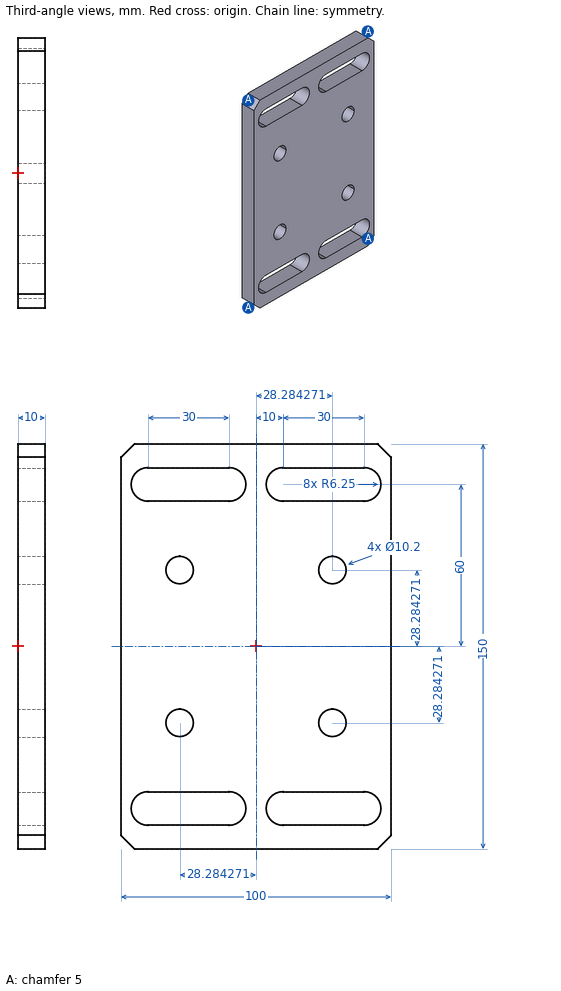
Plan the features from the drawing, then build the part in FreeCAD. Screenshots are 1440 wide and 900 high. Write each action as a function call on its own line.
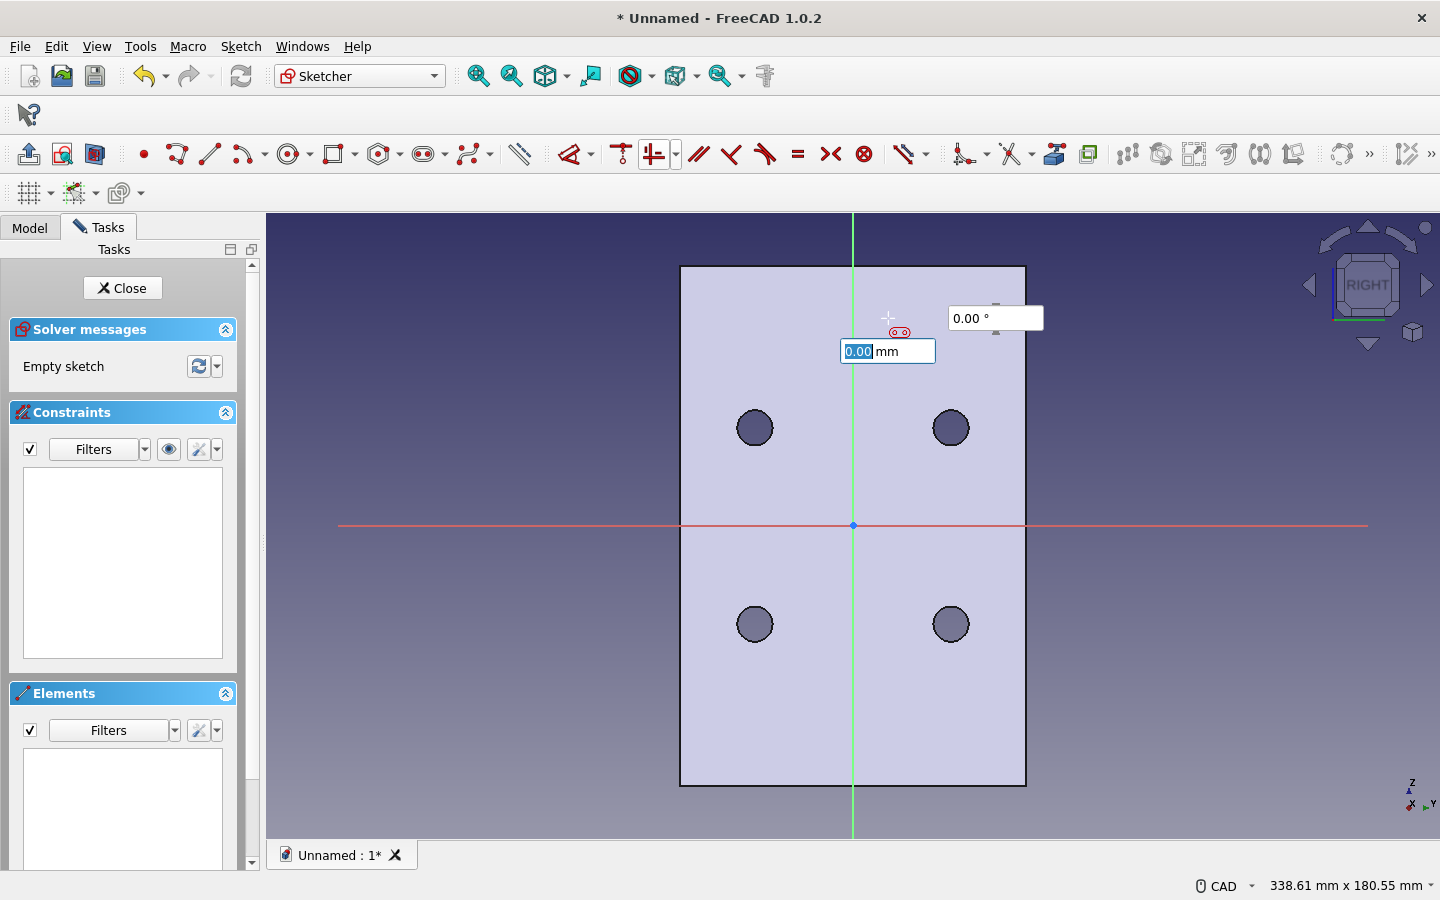
click(992, 318)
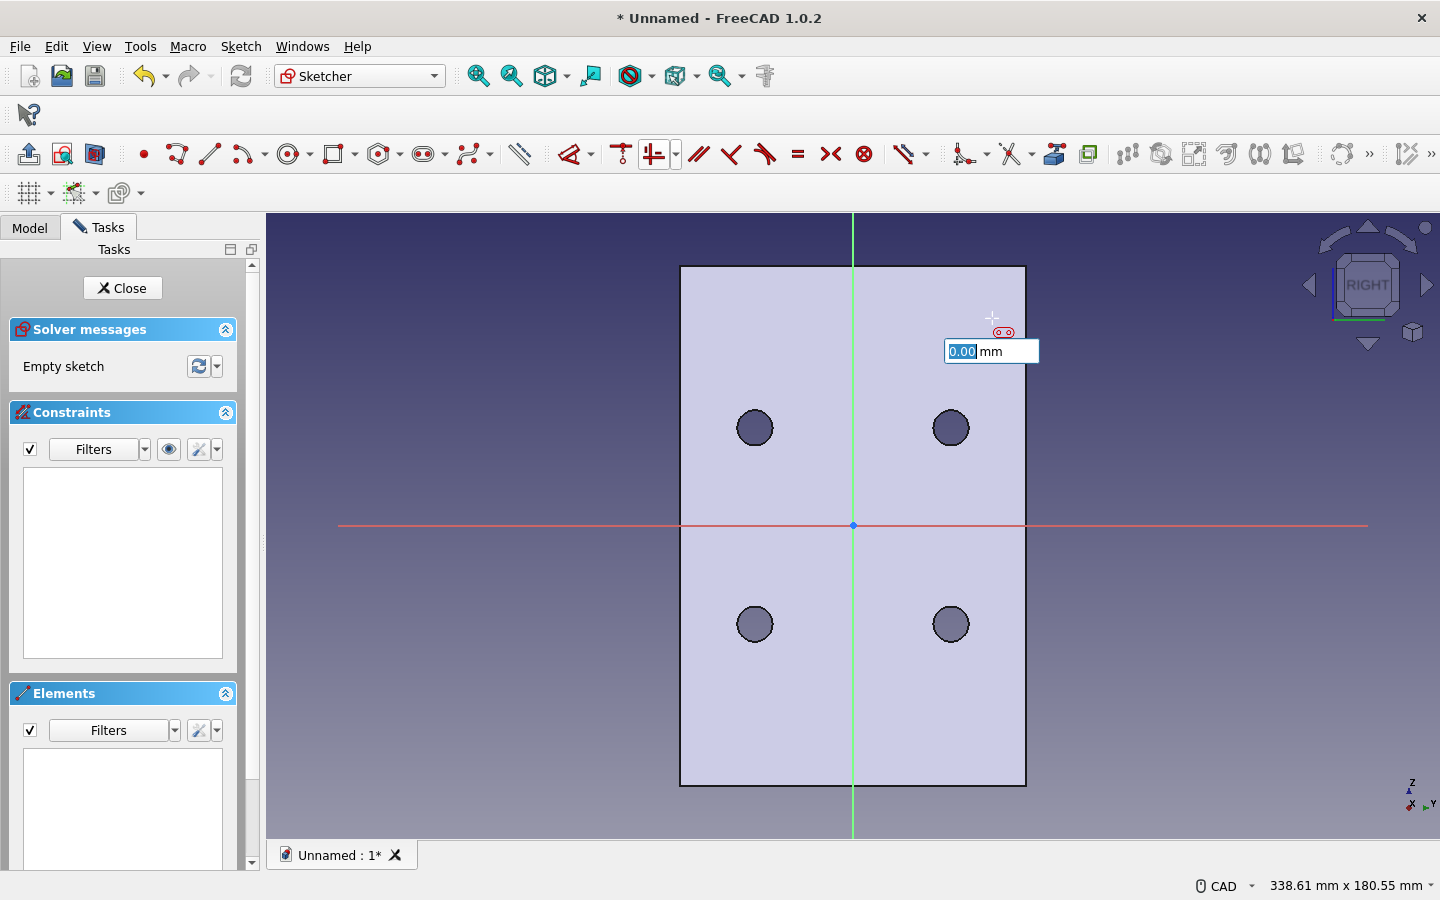
click(940, 340)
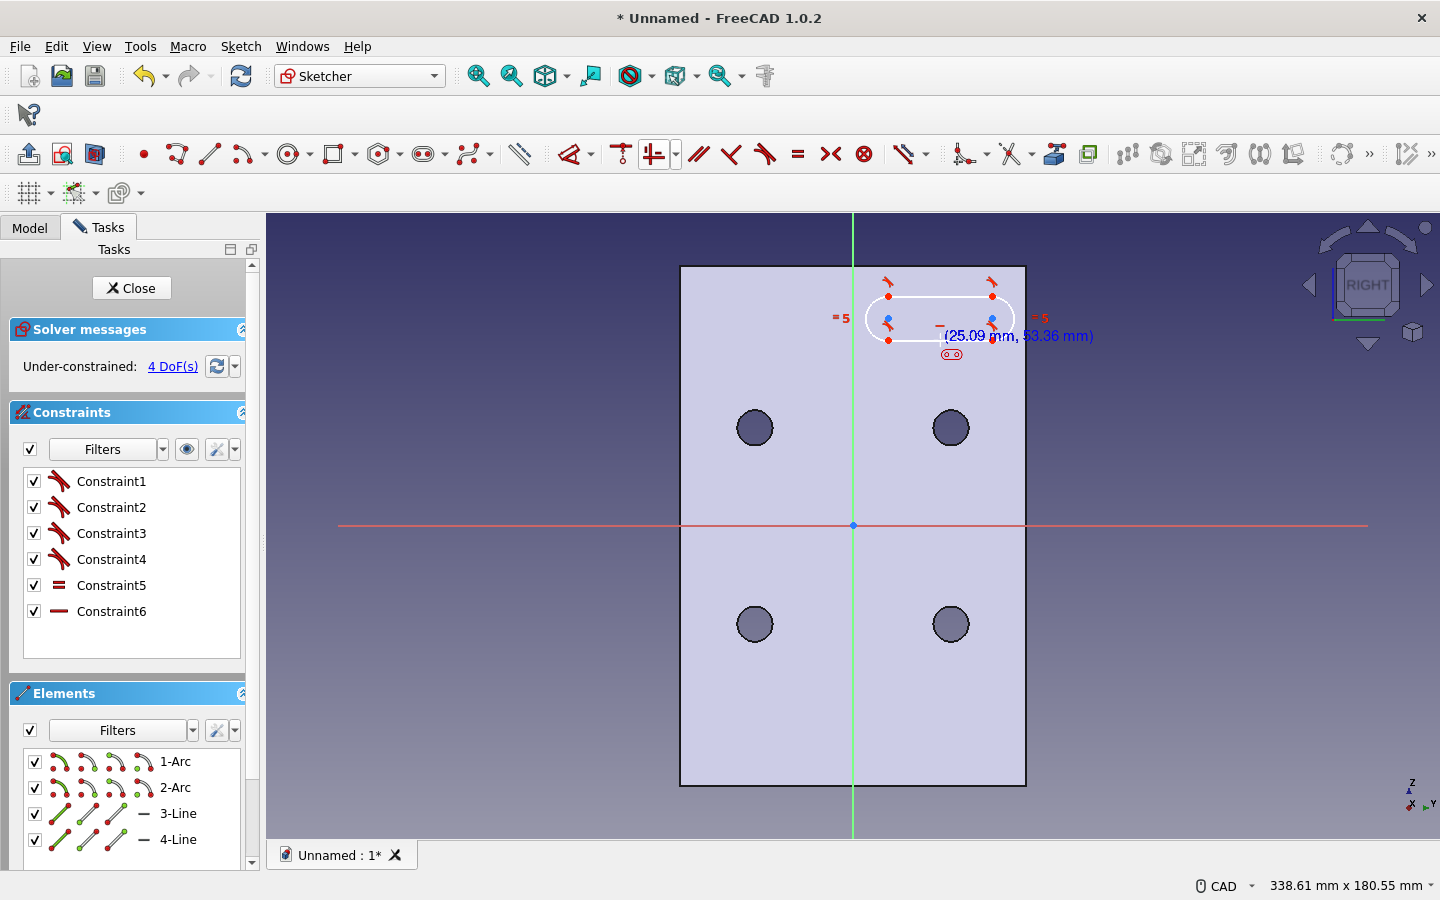
click(888, 734)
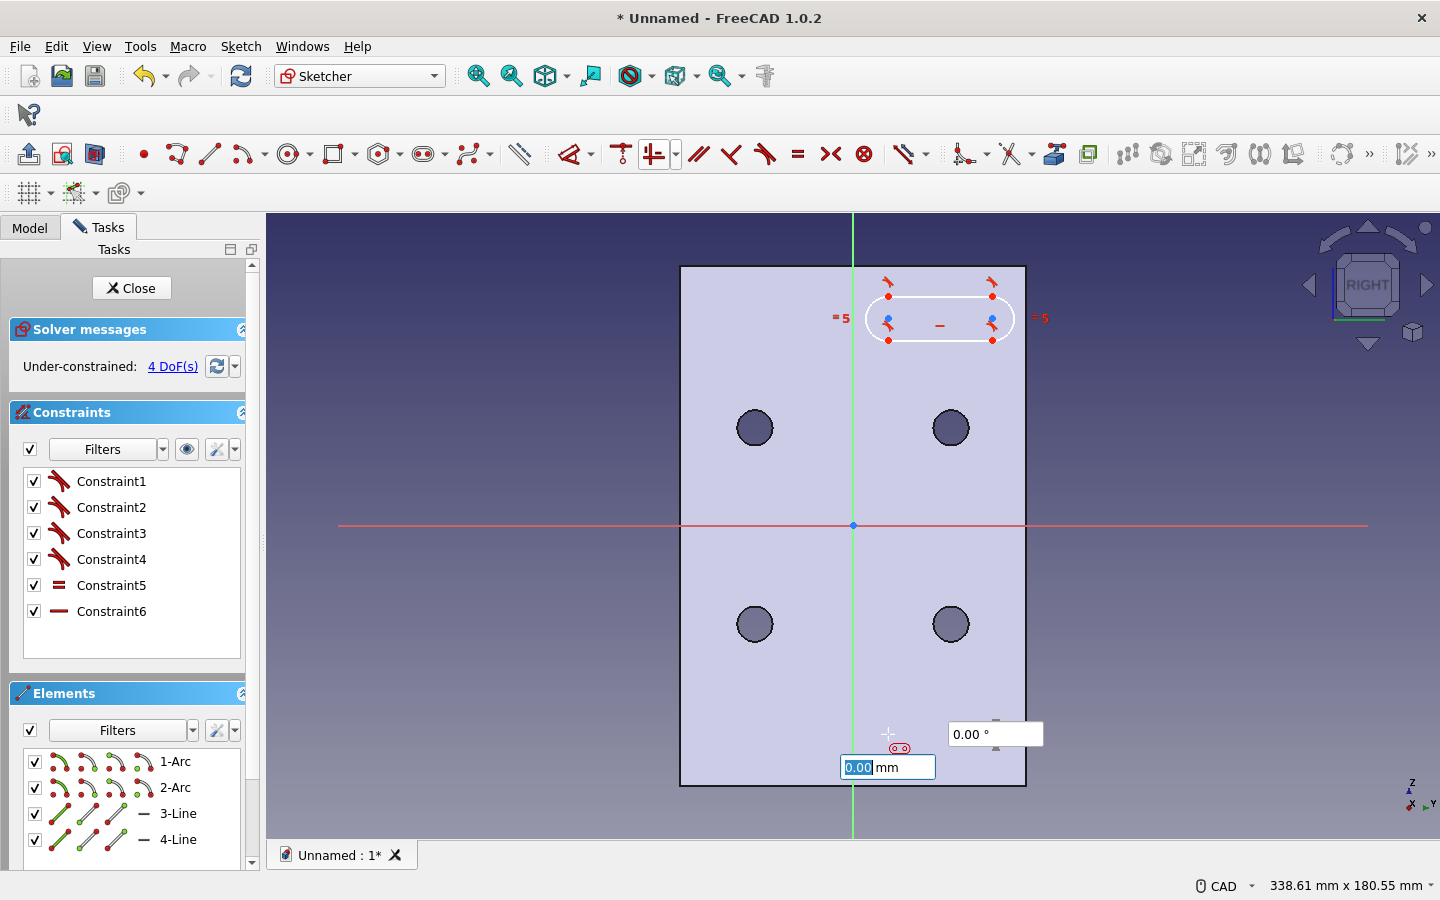
click(992, 734)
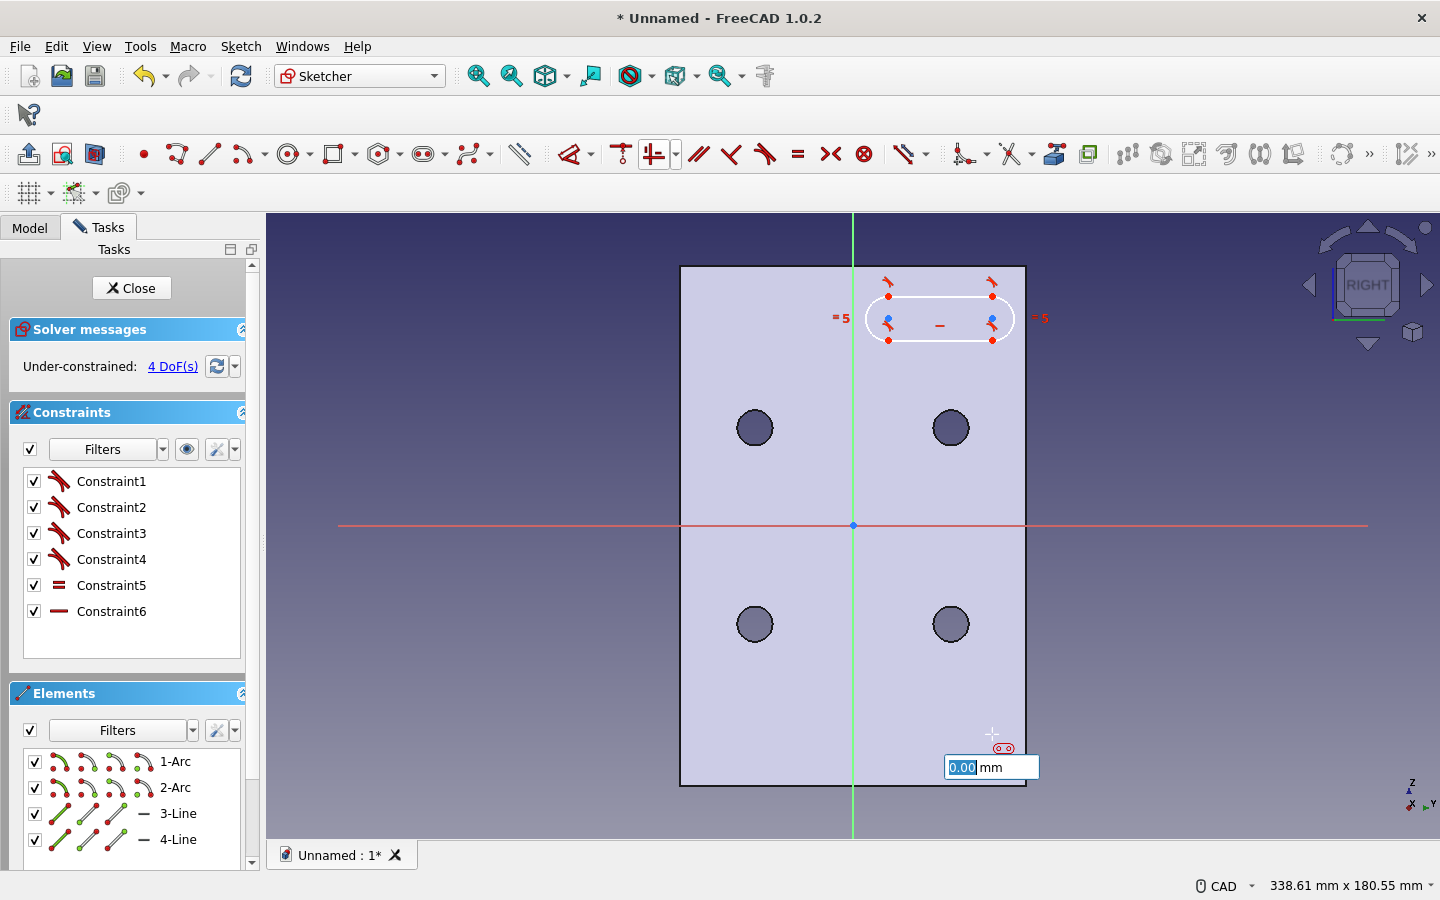
click(940, 712)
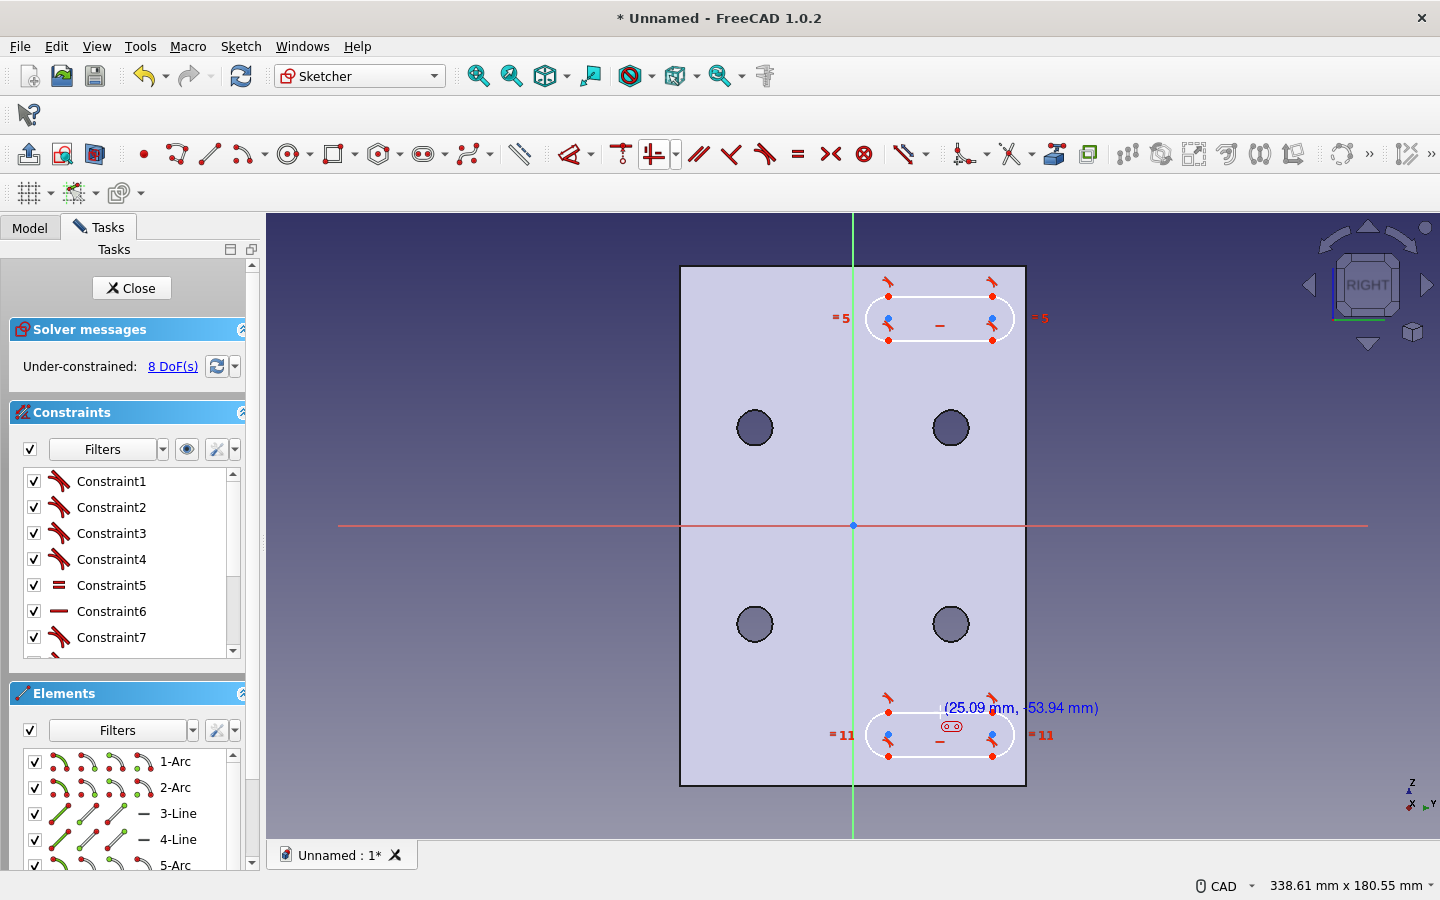
click(714, 318)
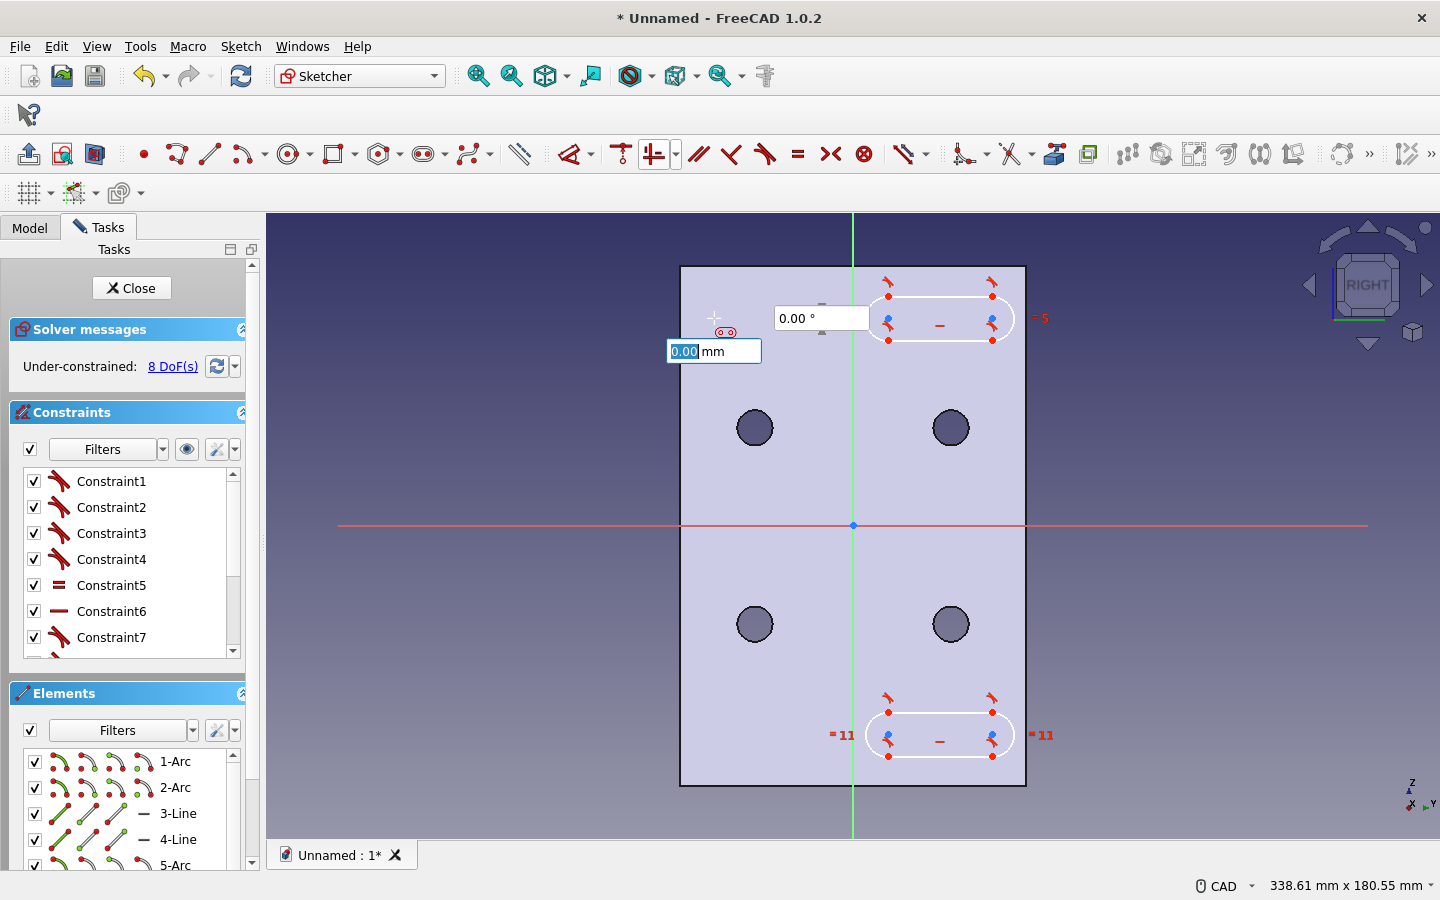
click(818, 318)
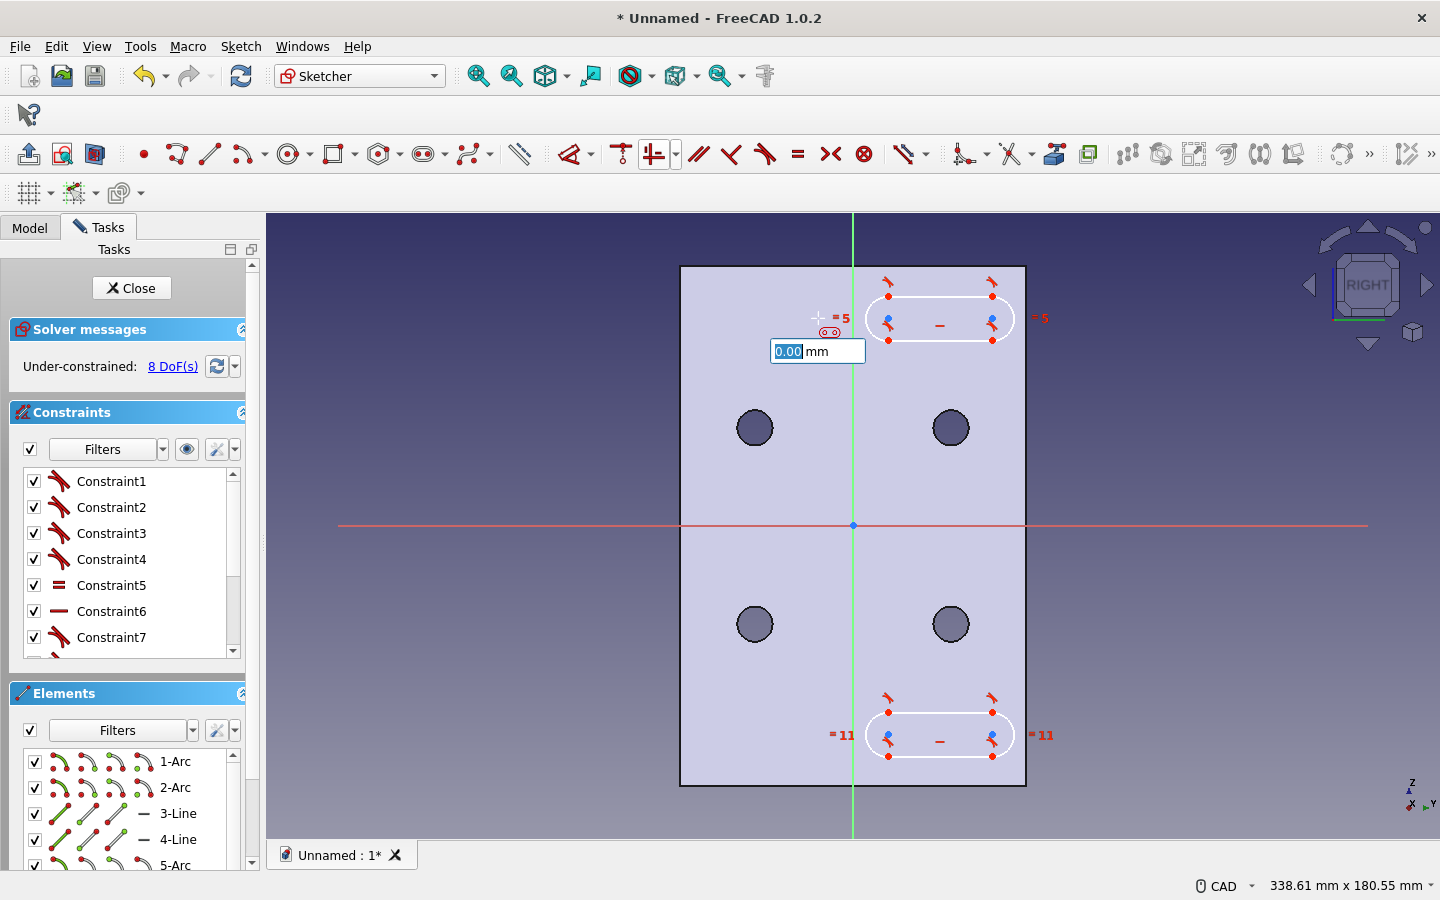
click(766, 340)